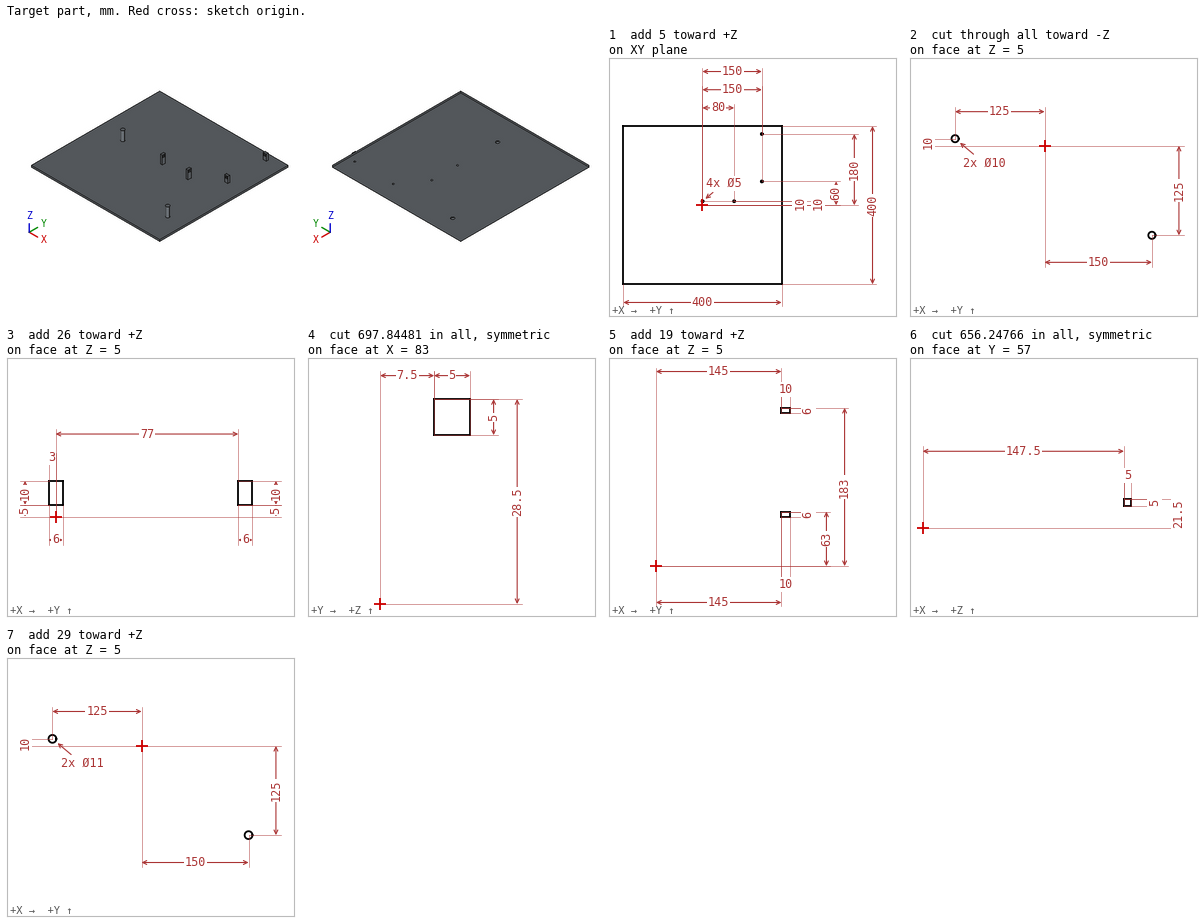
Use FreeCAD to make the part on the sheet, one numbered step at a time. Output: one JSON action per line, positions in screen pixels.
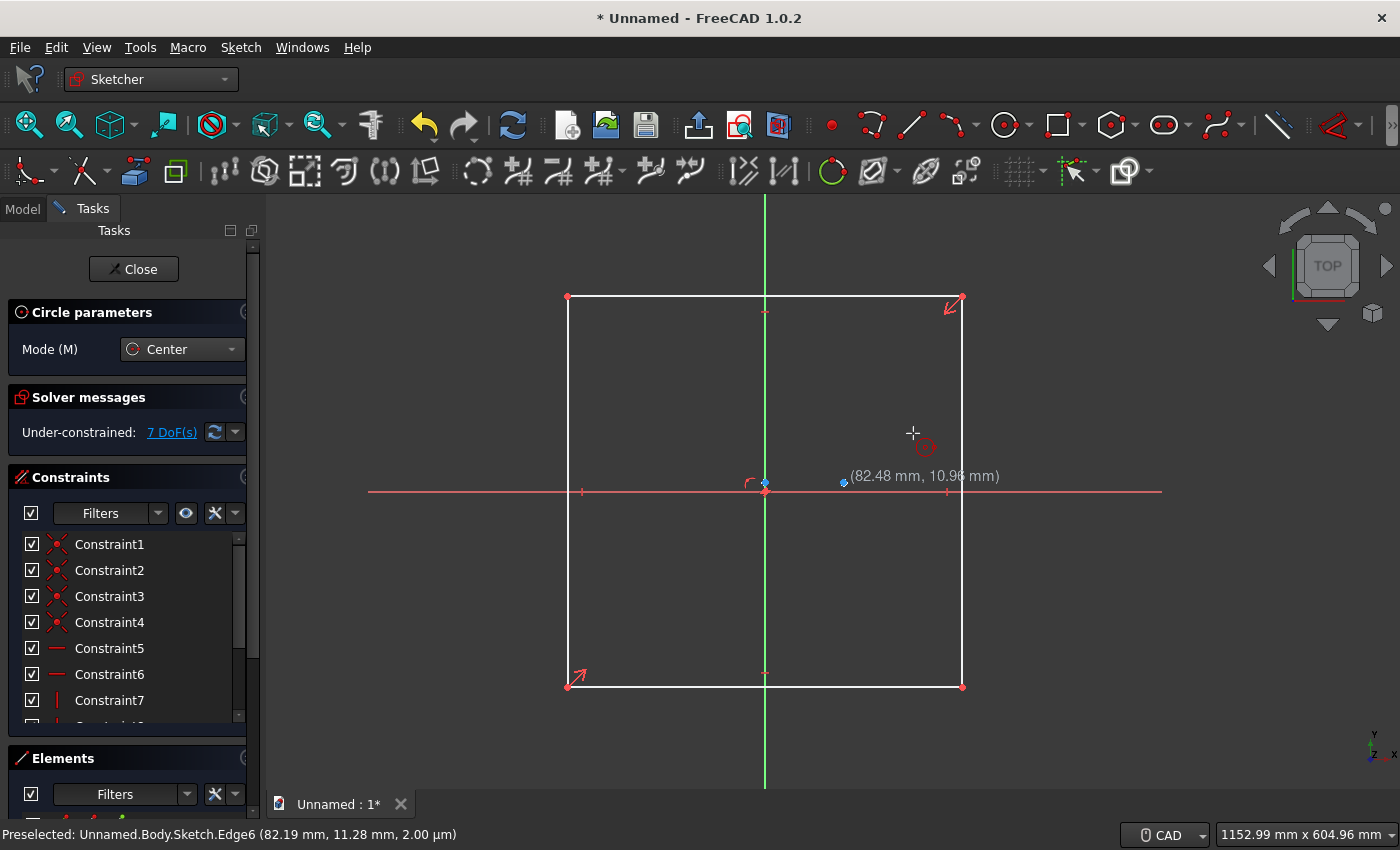
{"action": "left_click", "coordinate": [913, 433]}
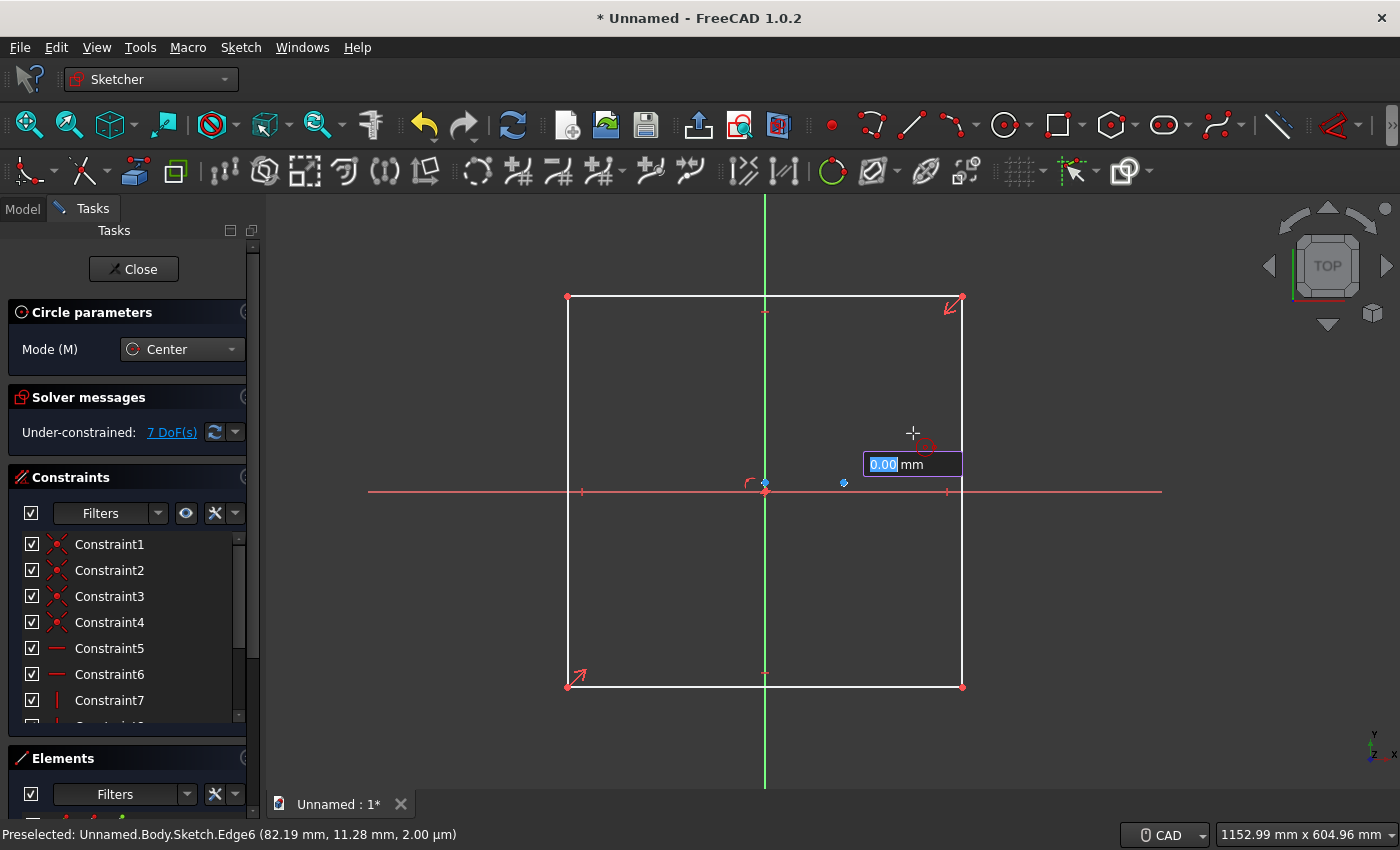
{"action": "scroll", "coordinate": [914, 431], "scroll_direction": "up", "scroll_amount": 10}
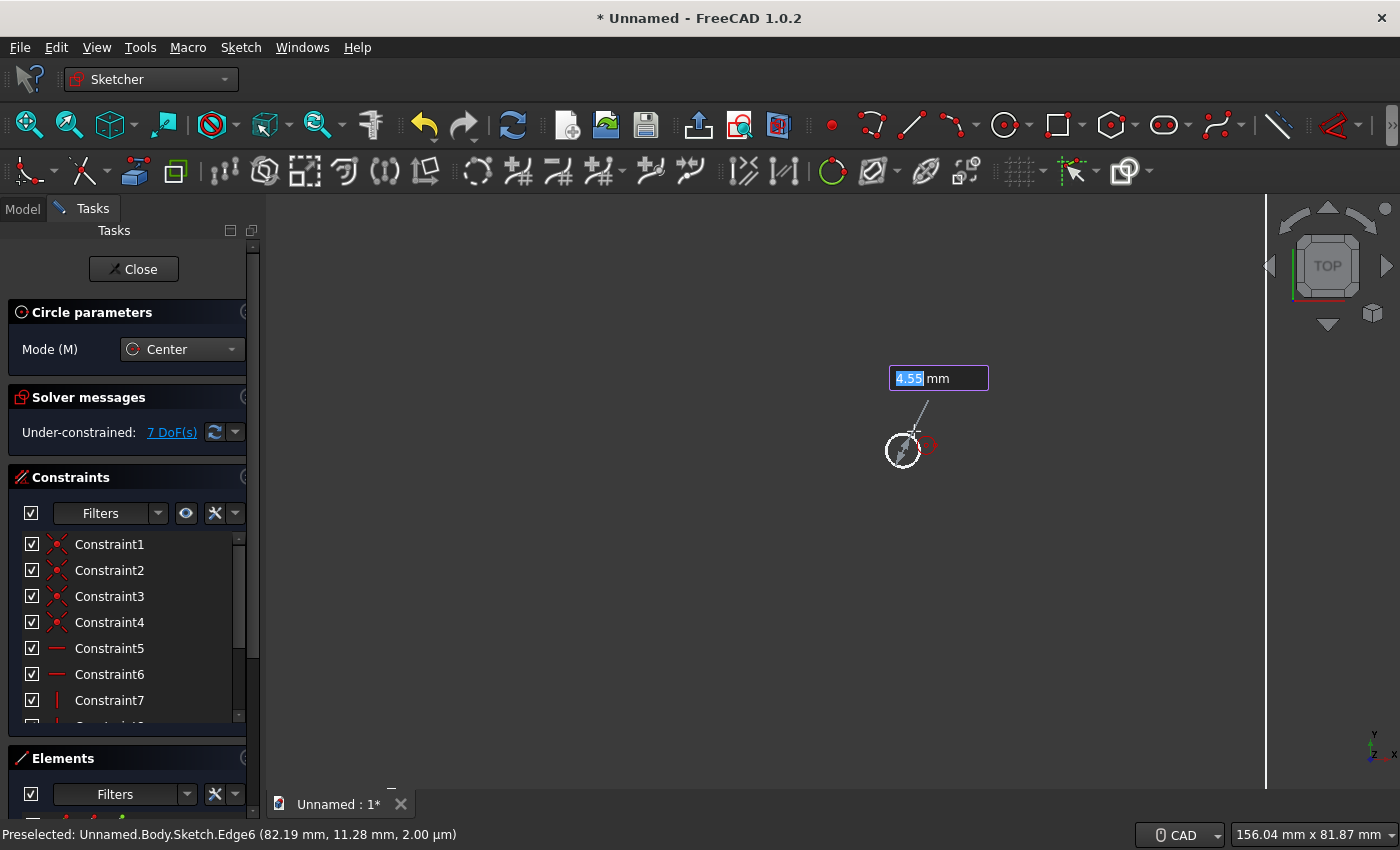
{"action": "left_click", "coordinate": [913, 429]}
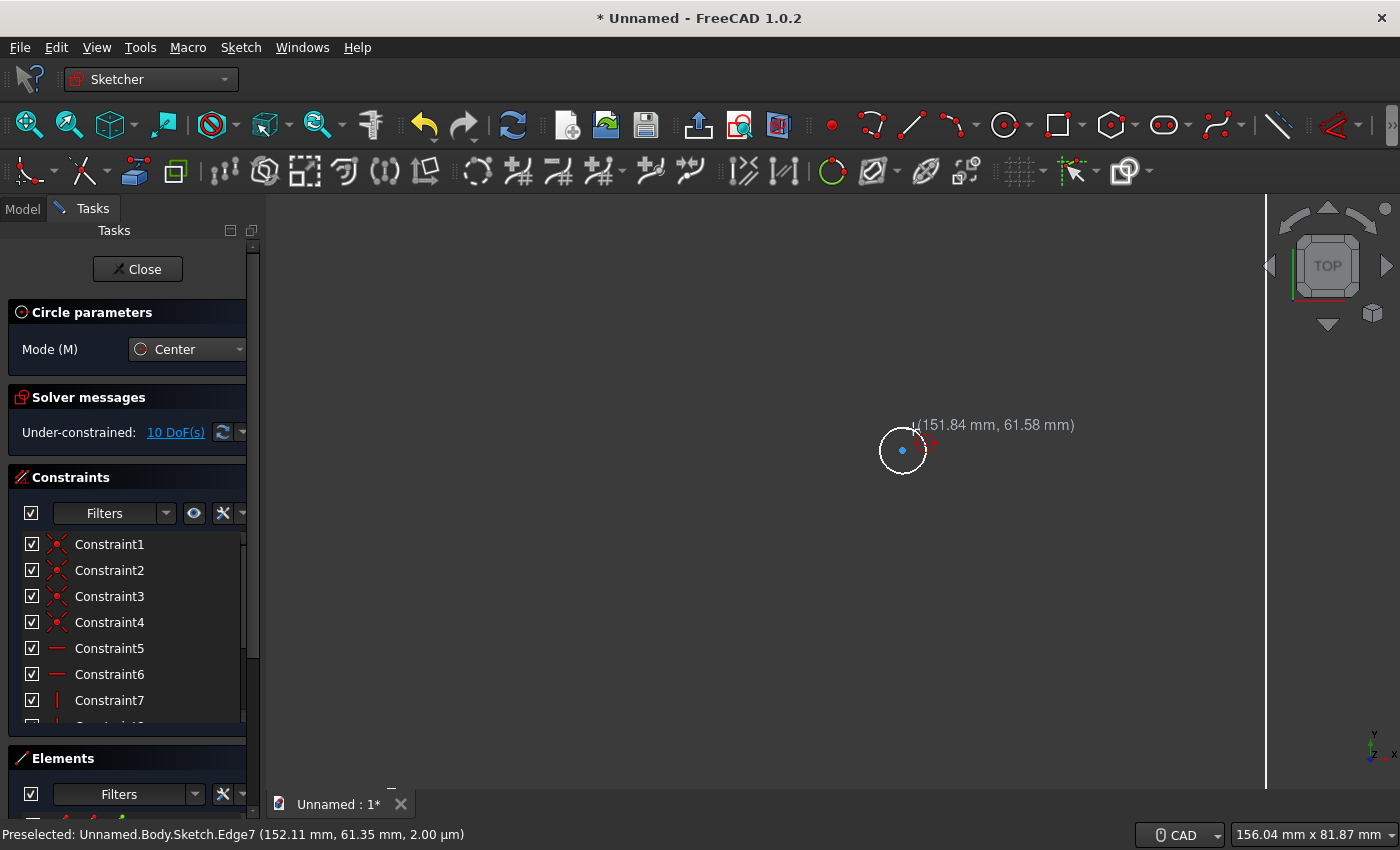
{"action": "scroll", "coordinate": [914, 431], "scroll_direction": "down", "scroll_amount": 10}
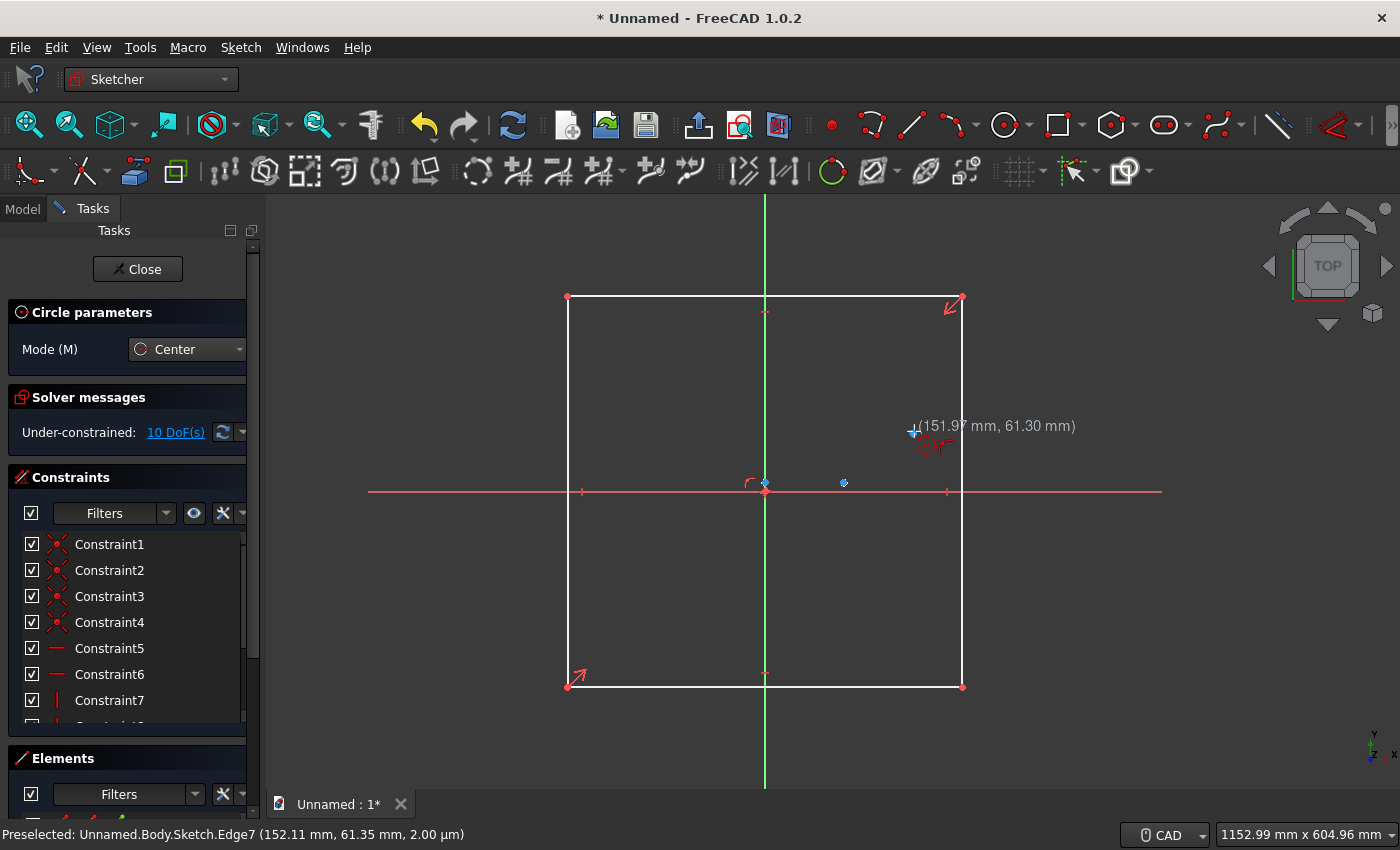
{"action": "scroll", "coordinate": [913, 315], "scroll_direction": "up", "scroll_amount": 12}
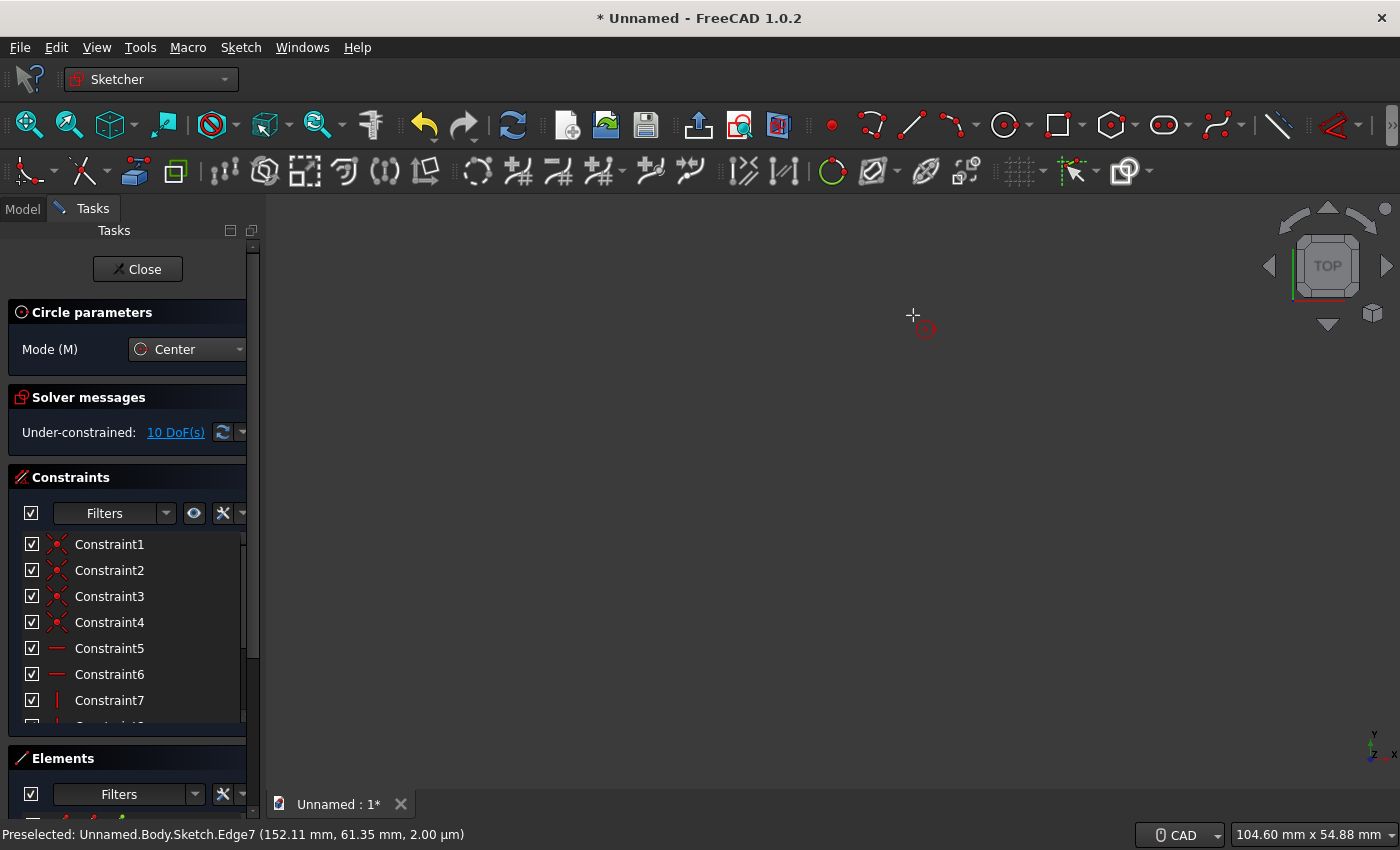
{"action": "scroll", "coordinate": [913, 315], "scroll_direction": "down", "scroll_amount": 12}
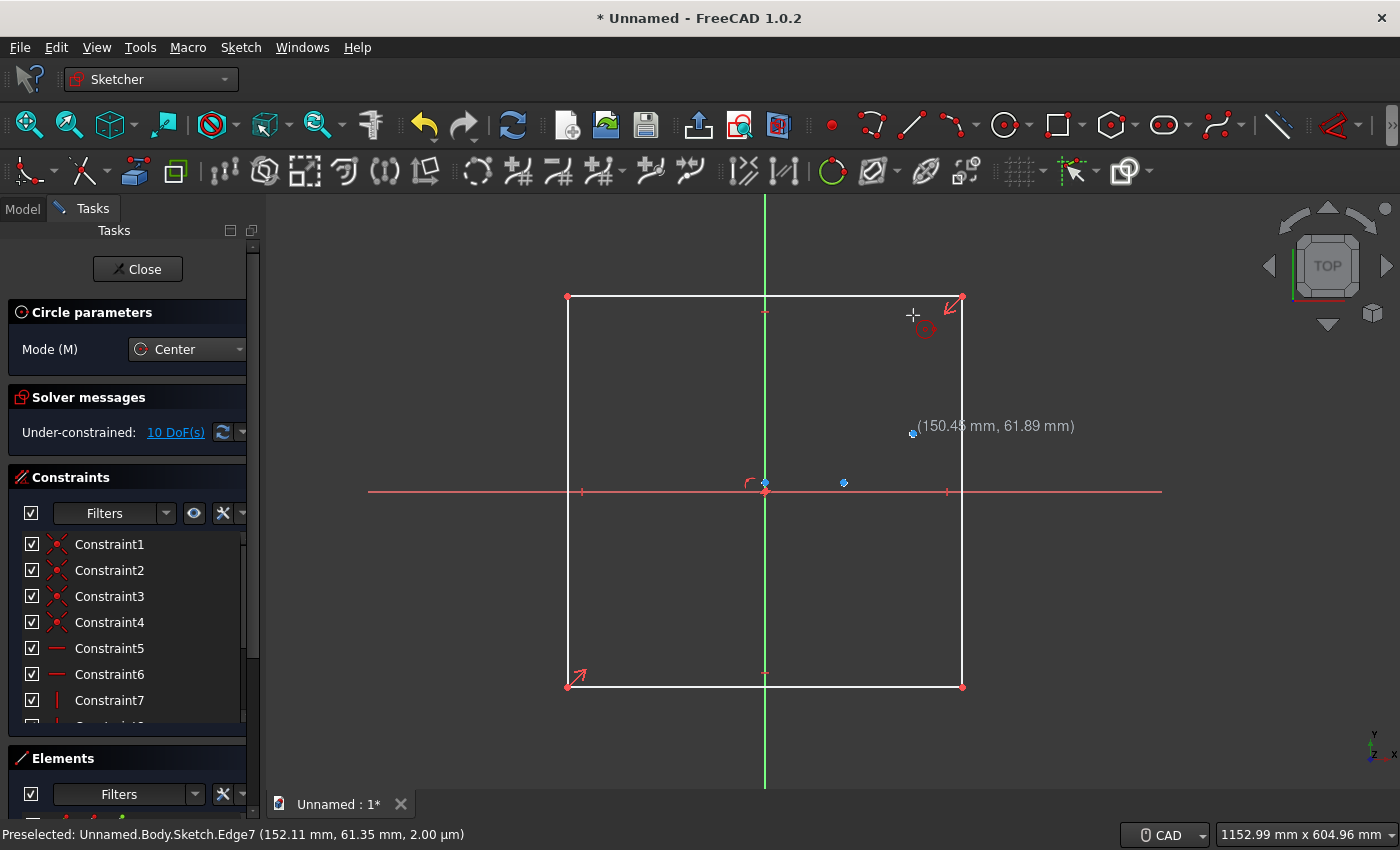
{"action": "left_click", "coordinate": [913, 315]}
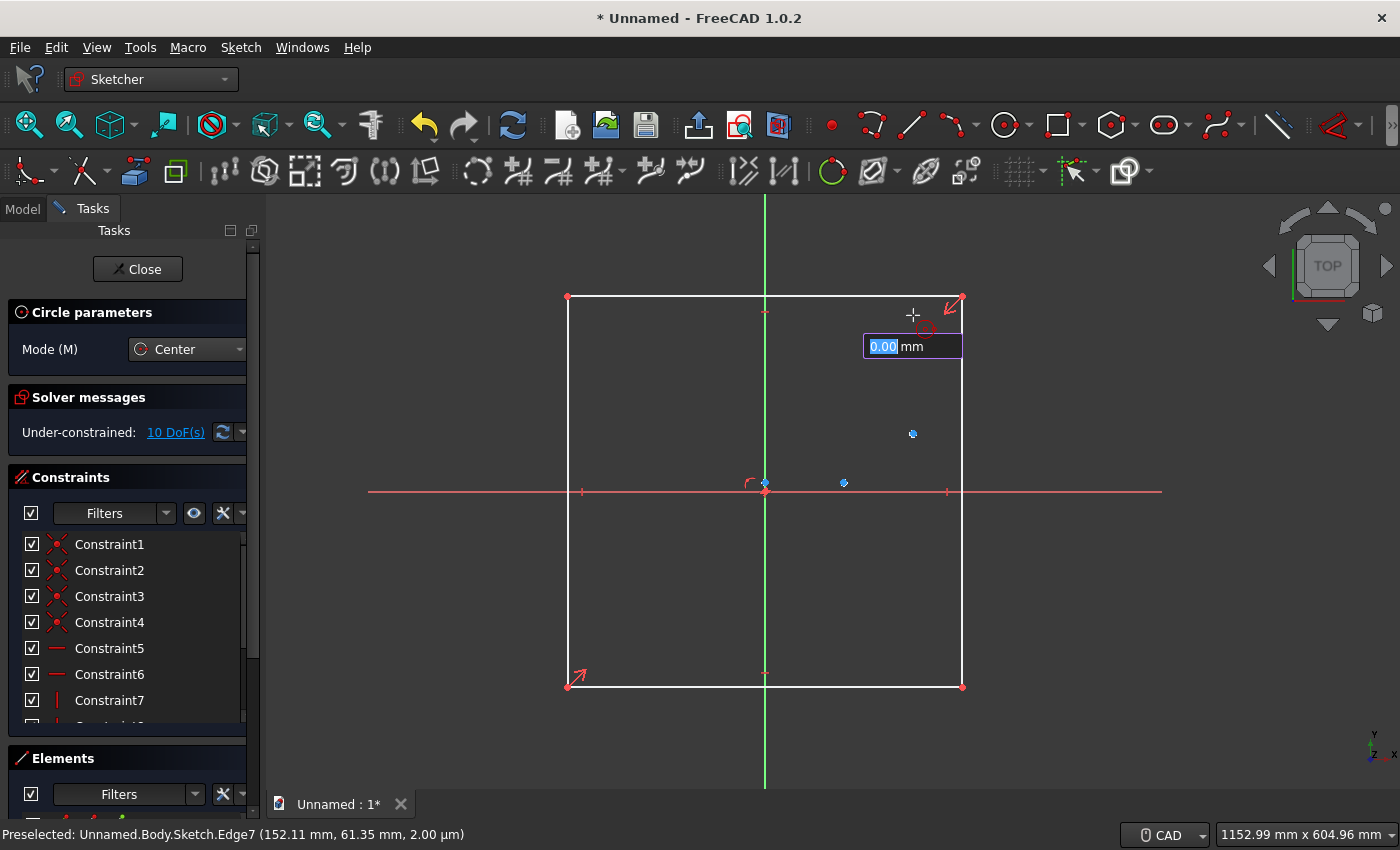
{"action": "scroll", "coordinate": [914, 313], "scroll_direction": "up", "scroll_amount": 10}